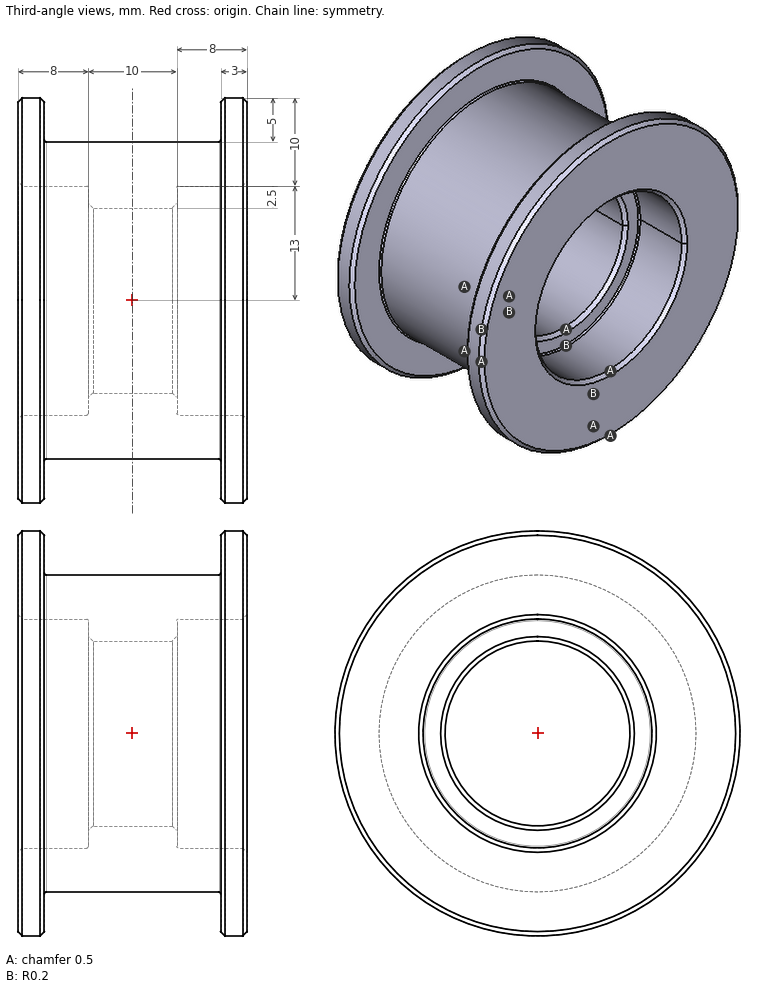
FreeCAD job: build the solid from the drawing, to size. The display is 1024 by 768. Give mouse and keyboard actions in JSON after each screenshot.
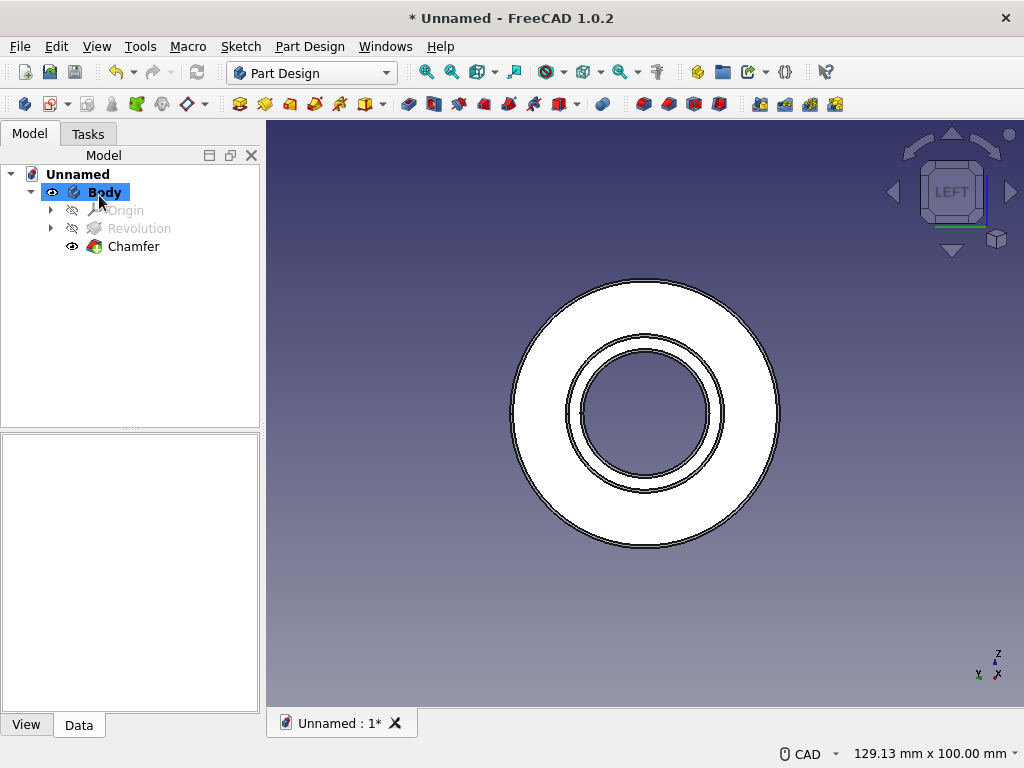
{"action": "key", "text": "0"}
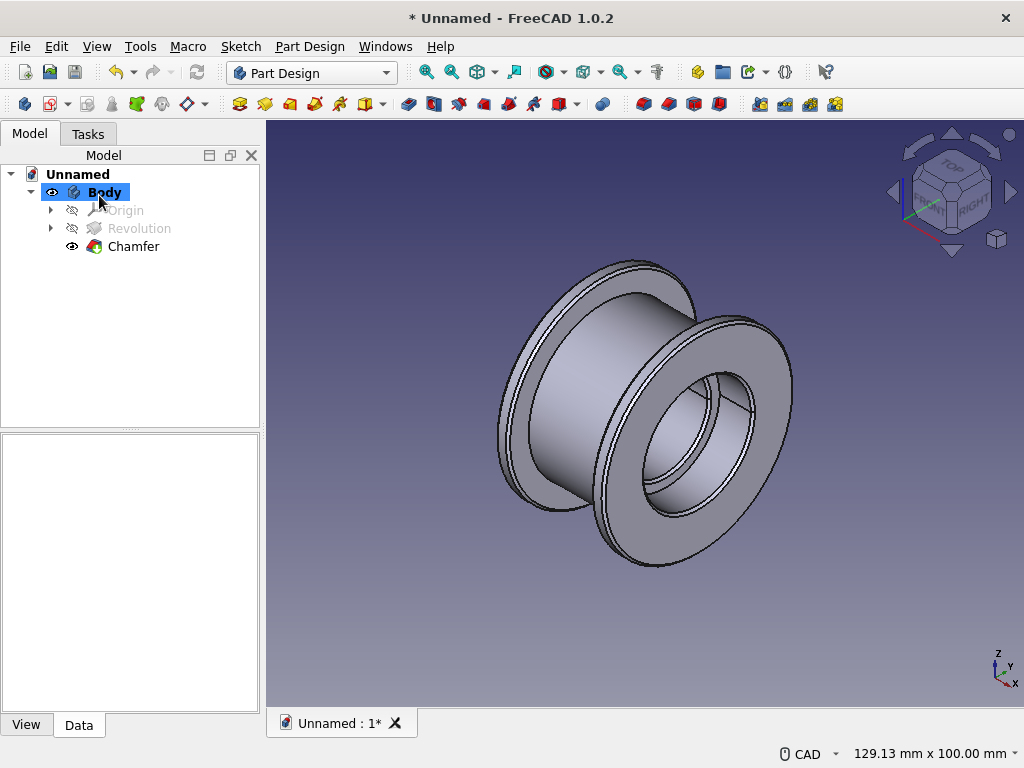
{"action": "key", "text": "2"}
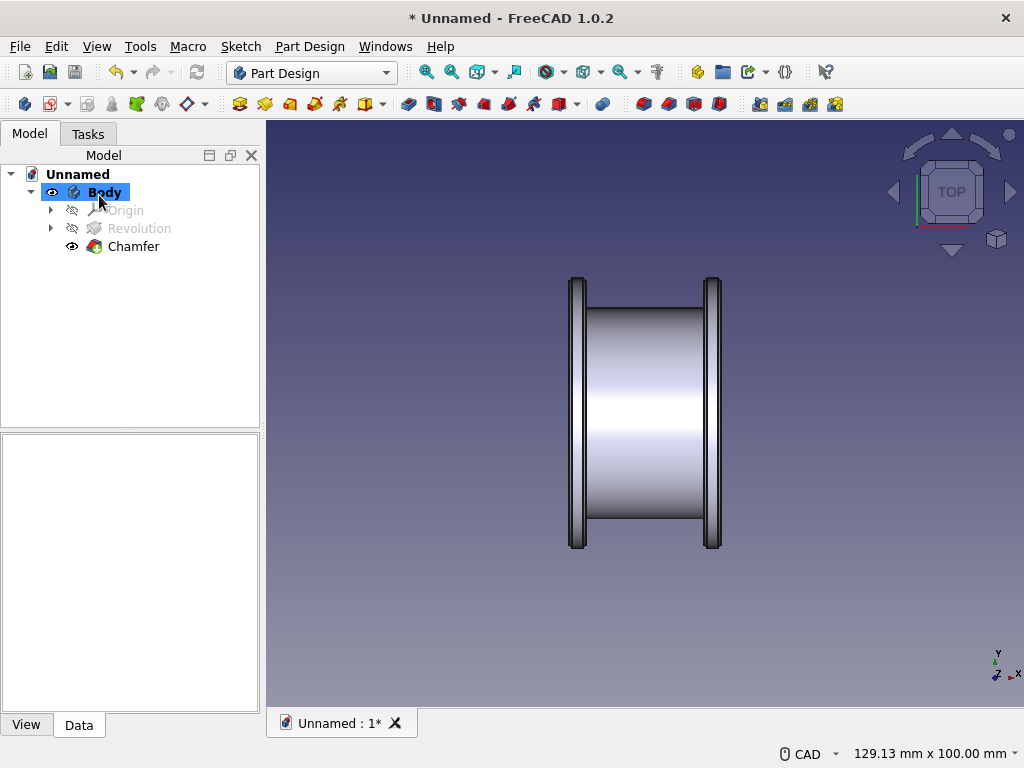
{"action": "key", "text": "1"}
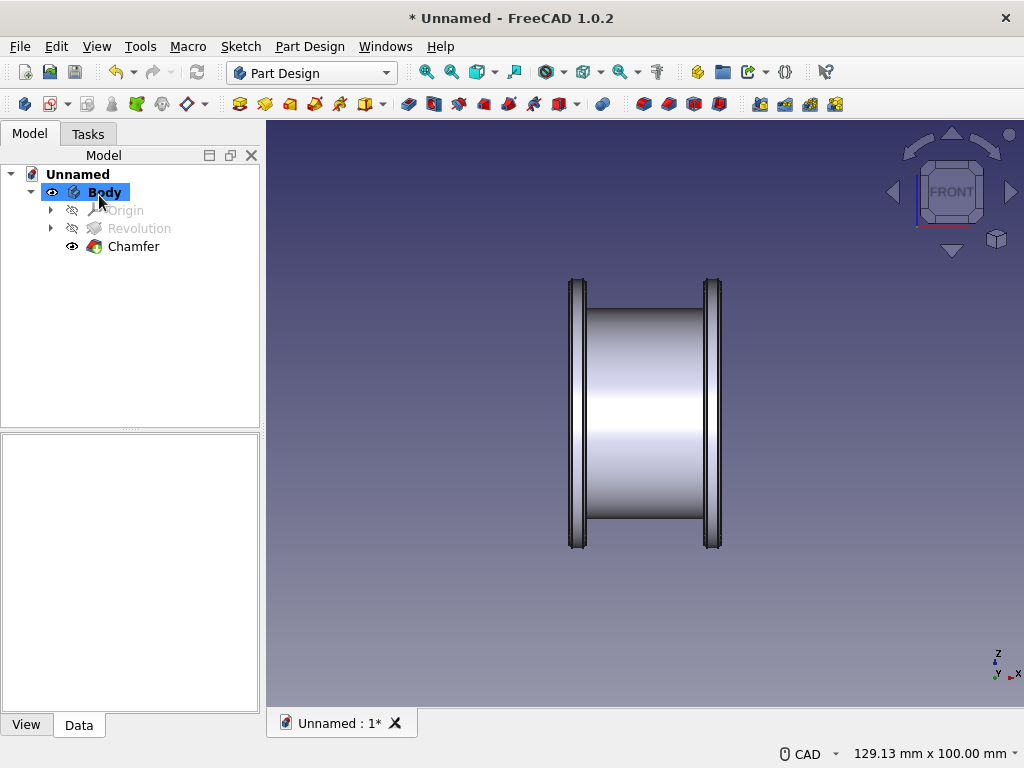
{"action": "key", "text": "3"}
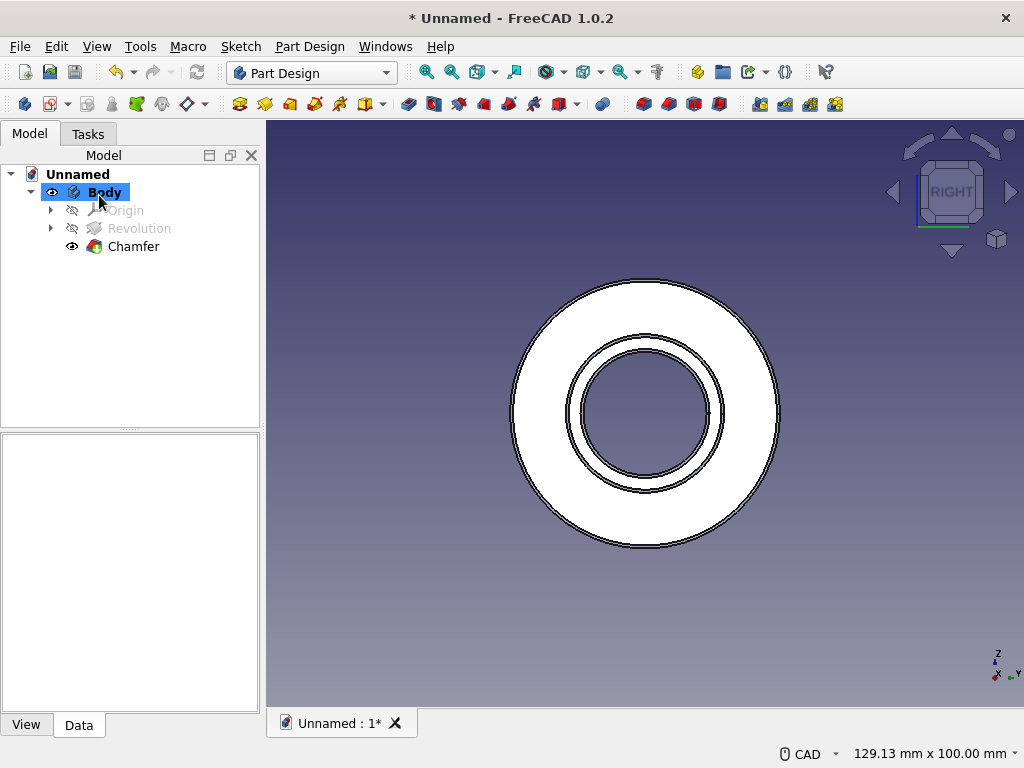
{"action": "key", "text": "5"}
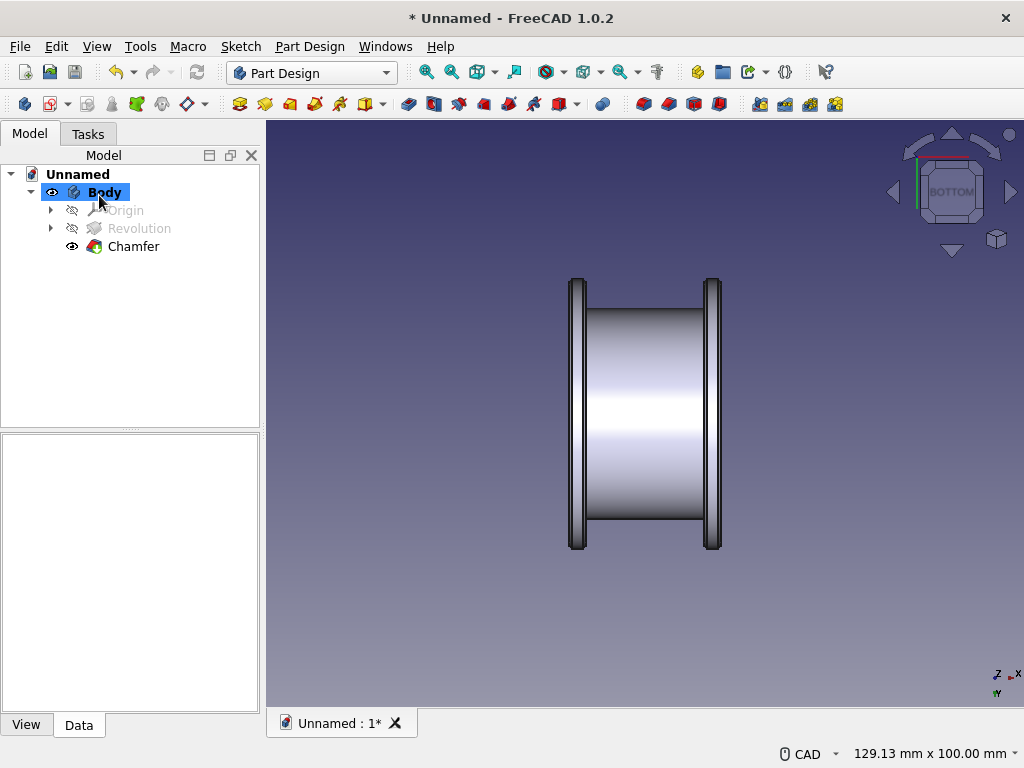
{"action": "key", "text": "4"}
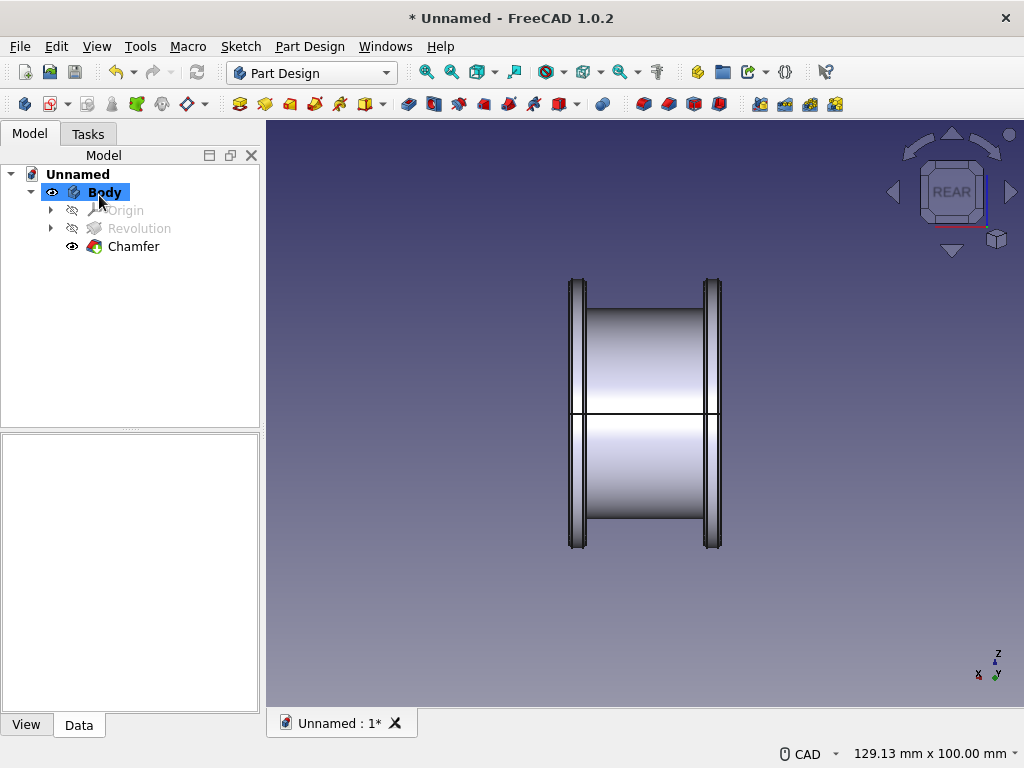
{"action": "key", "text": "6"}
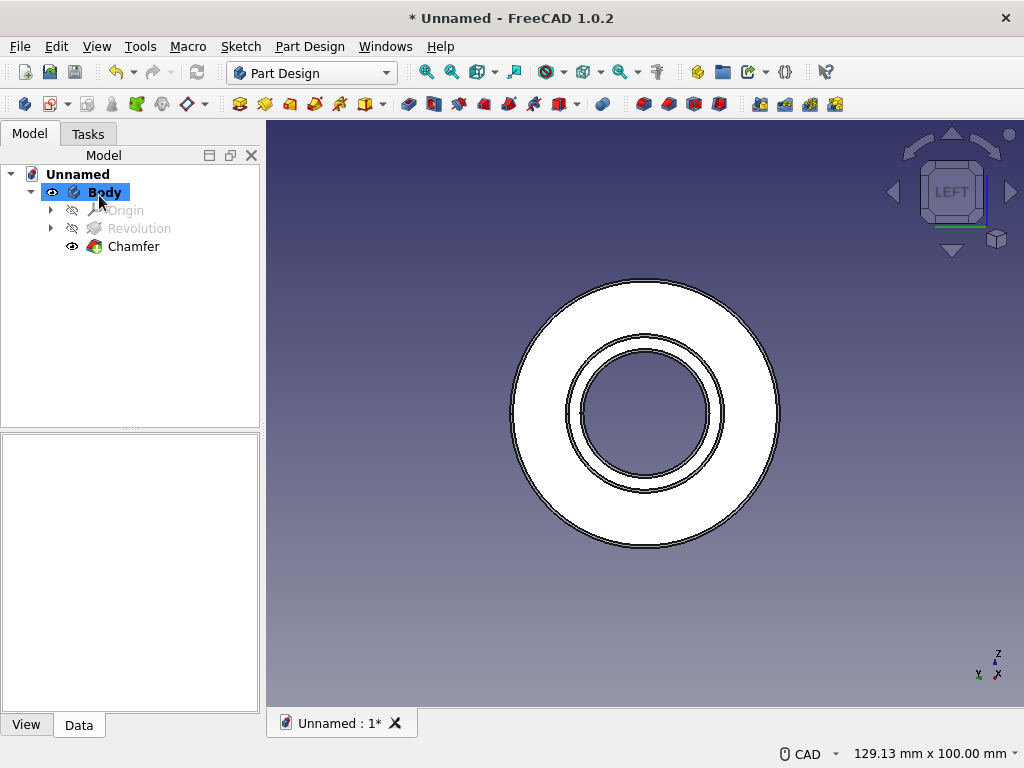
{"action": "key", "text": "v 3"}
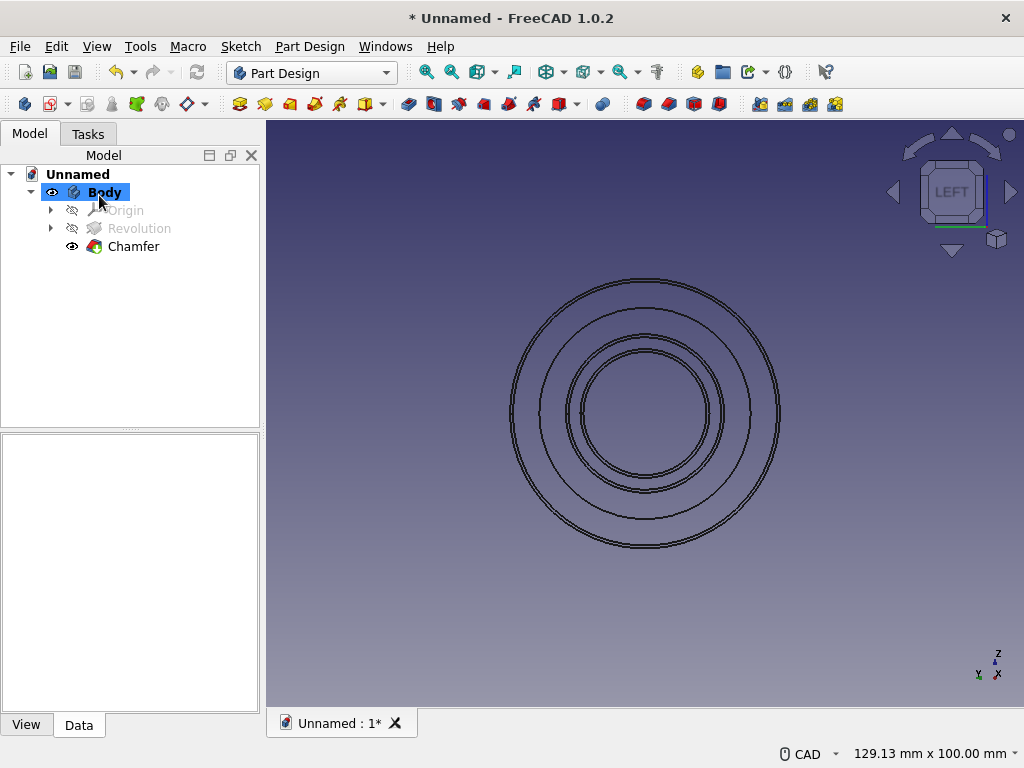
{"action": "key", "text": "0"}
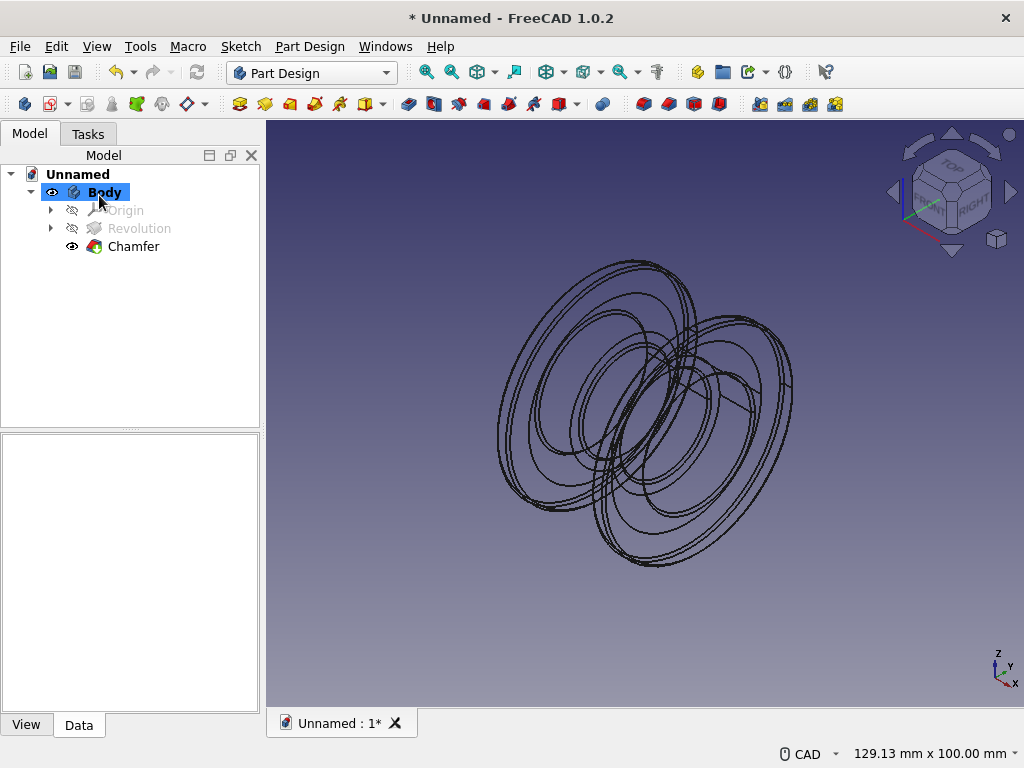
{"action": "left_click", "coordinate": [626, 522]}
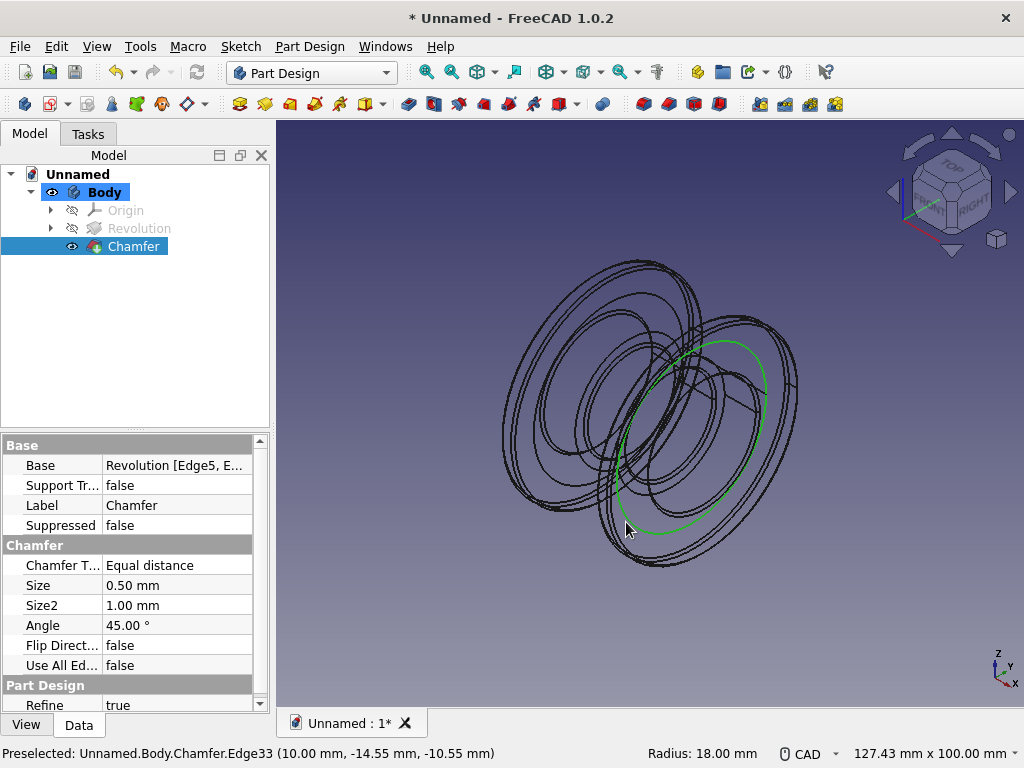
{"action": "left_click", "coordinate": [534, 432], "text": "ctrl"}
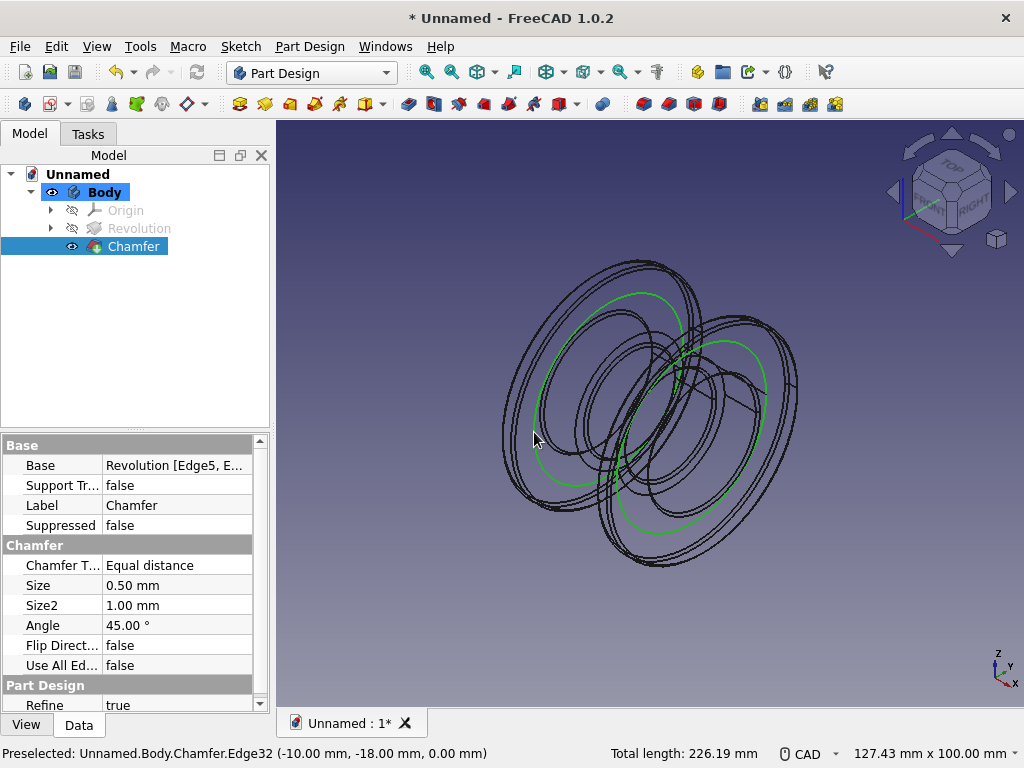
{"action": "left_click", "coordinate": [575, 432], "text": "ctrl"}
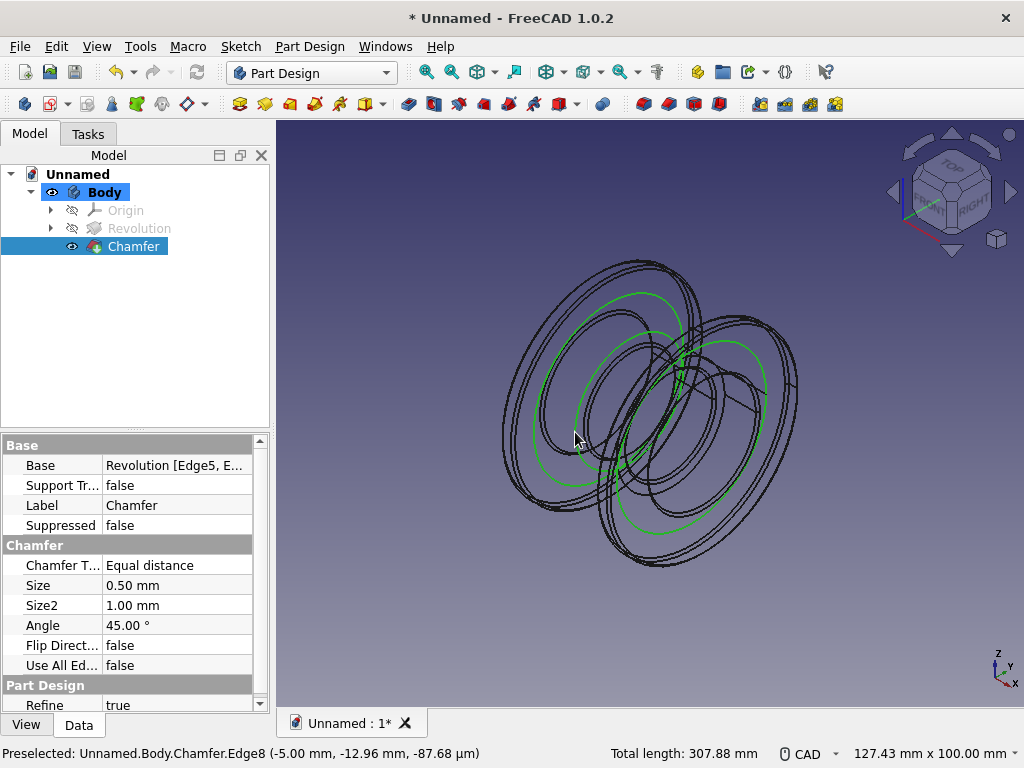
{"action": "left_click", "coordinate": [627, 486], "text": "ctrl"}